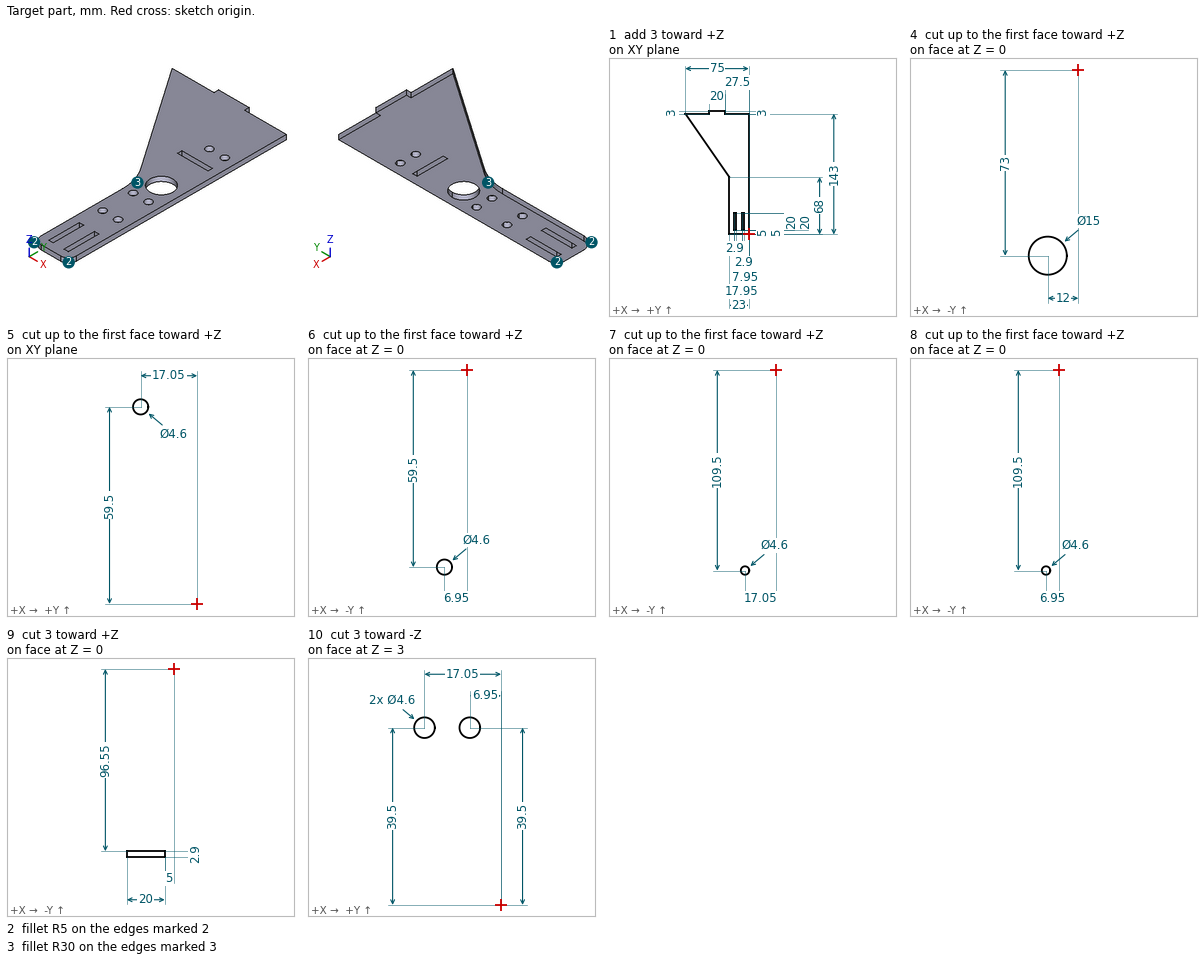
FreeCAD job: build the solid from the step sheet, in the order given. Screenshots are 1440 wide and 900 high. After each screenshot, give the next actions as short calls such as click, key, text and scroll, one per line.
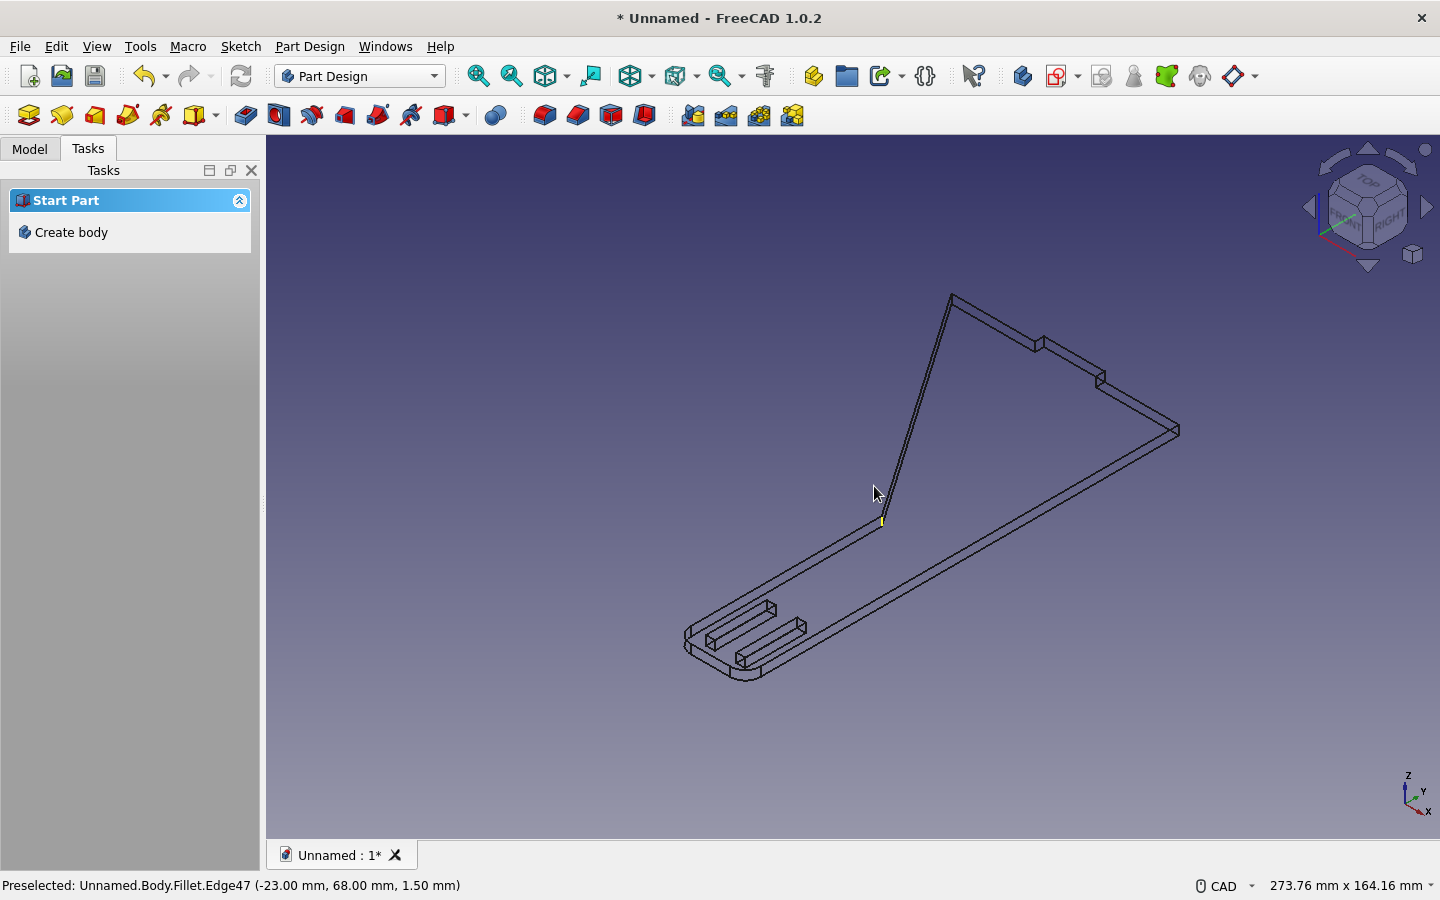
click(882, 523)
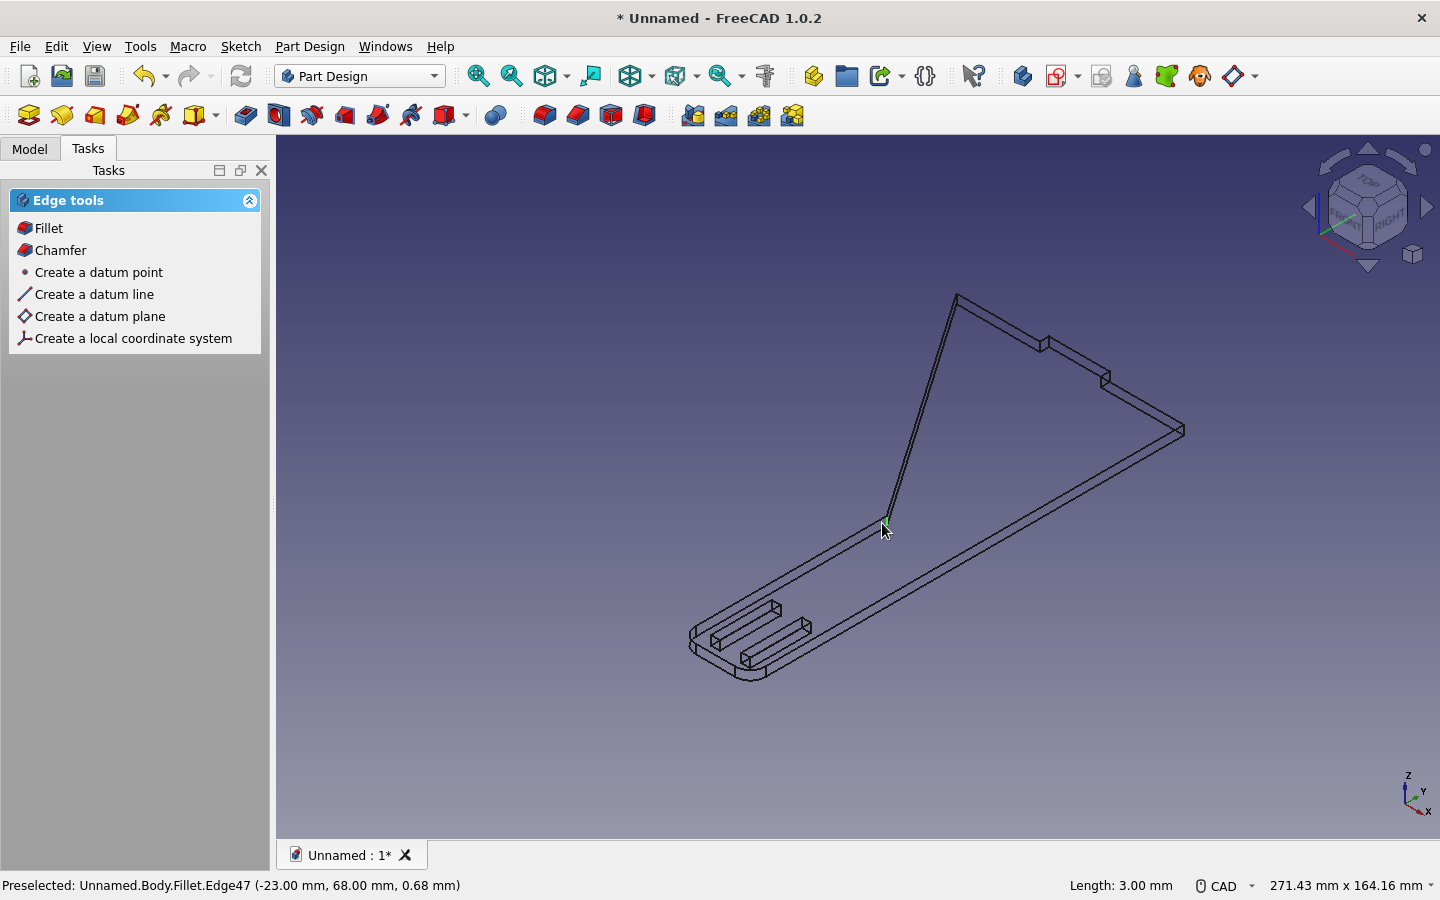
key(v)
key(1)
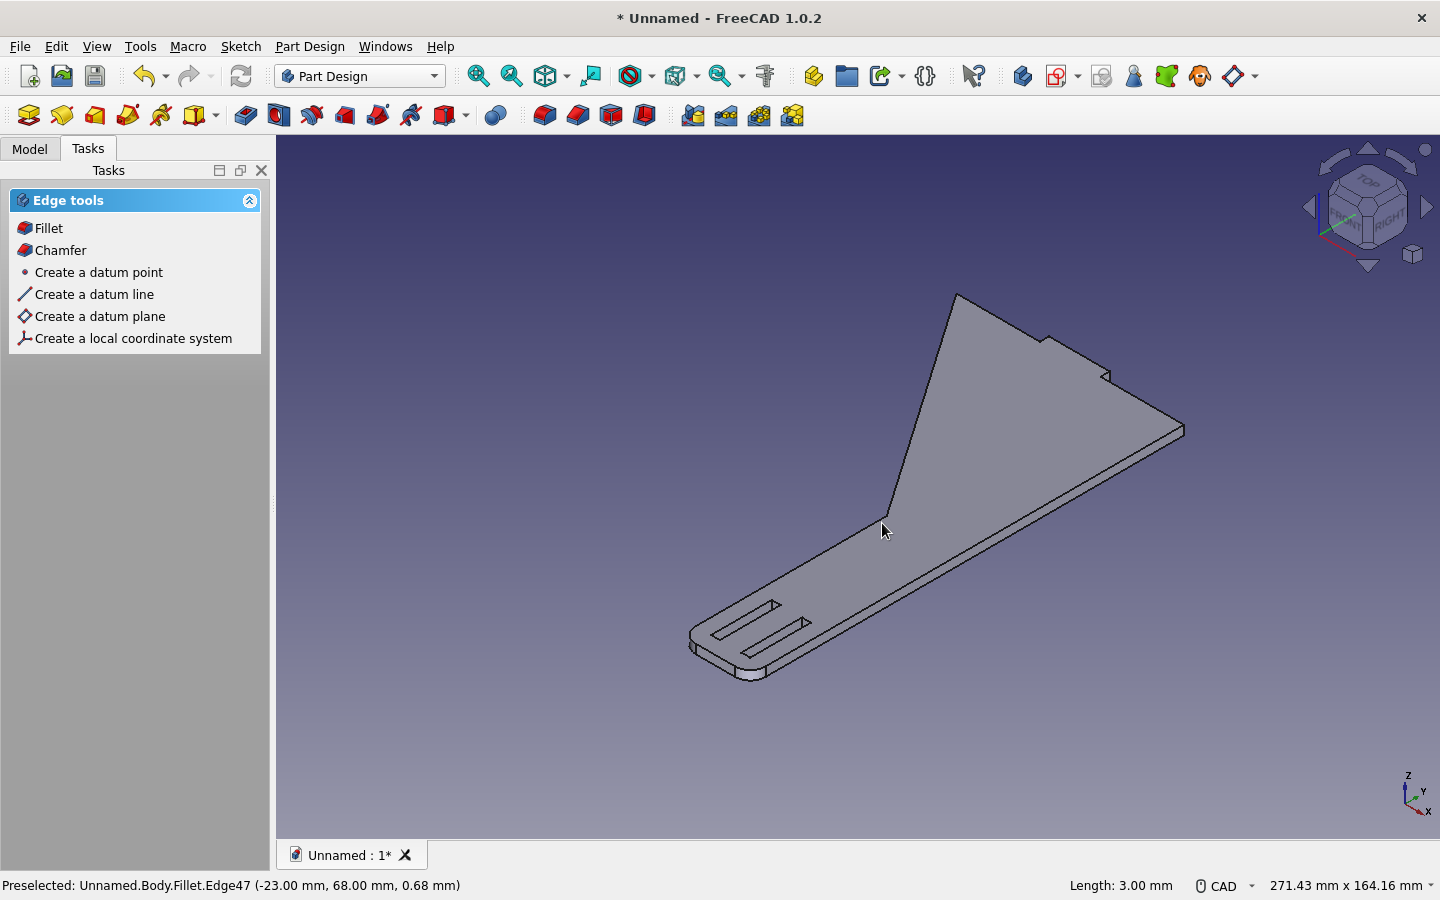
click(545, 116)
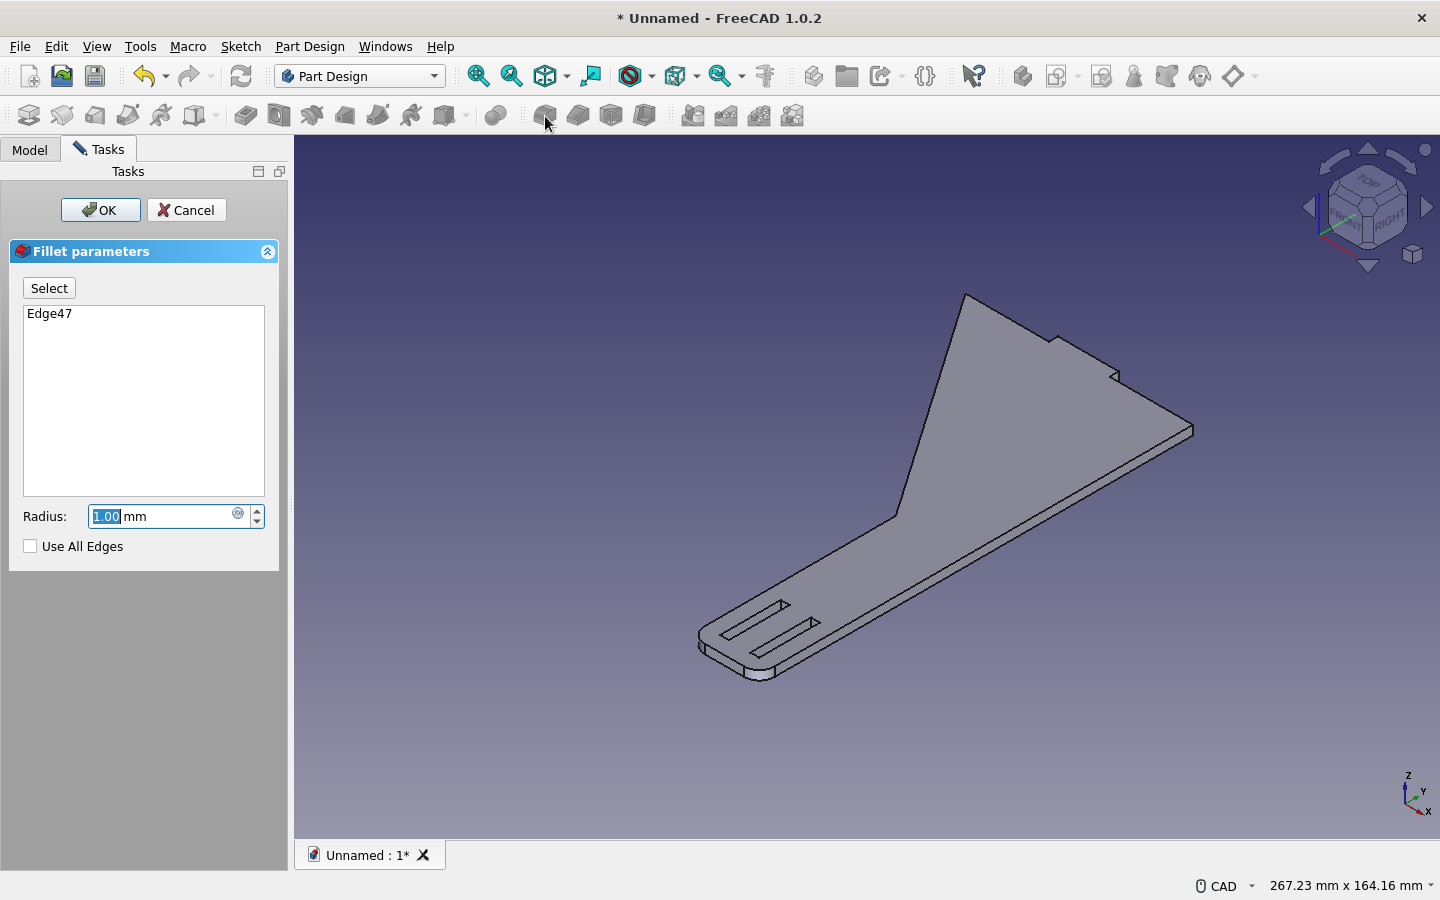
text(30)
key(Tab)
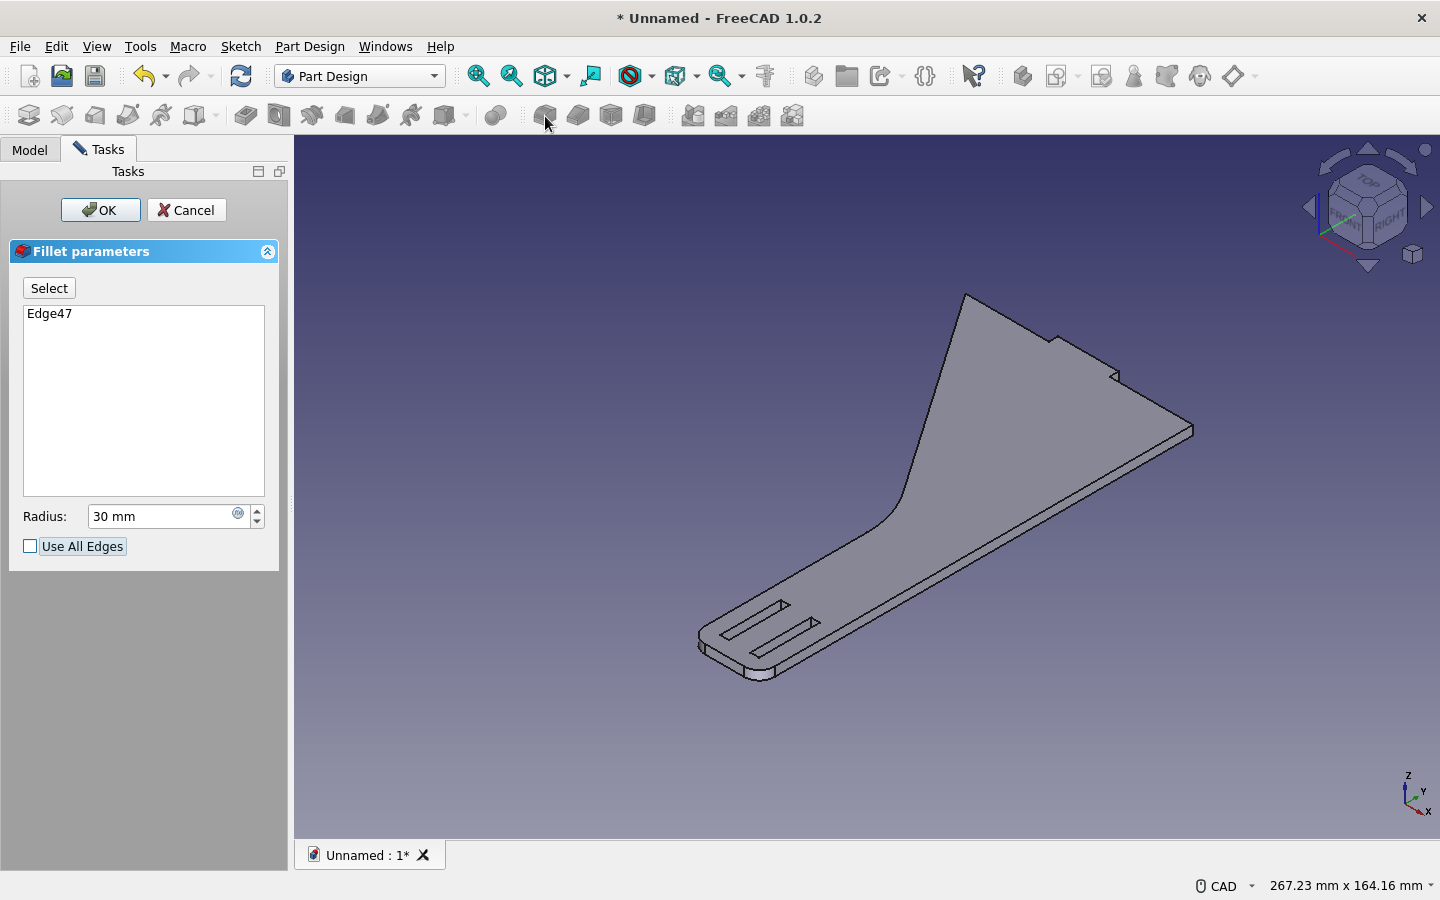
click(101, 210)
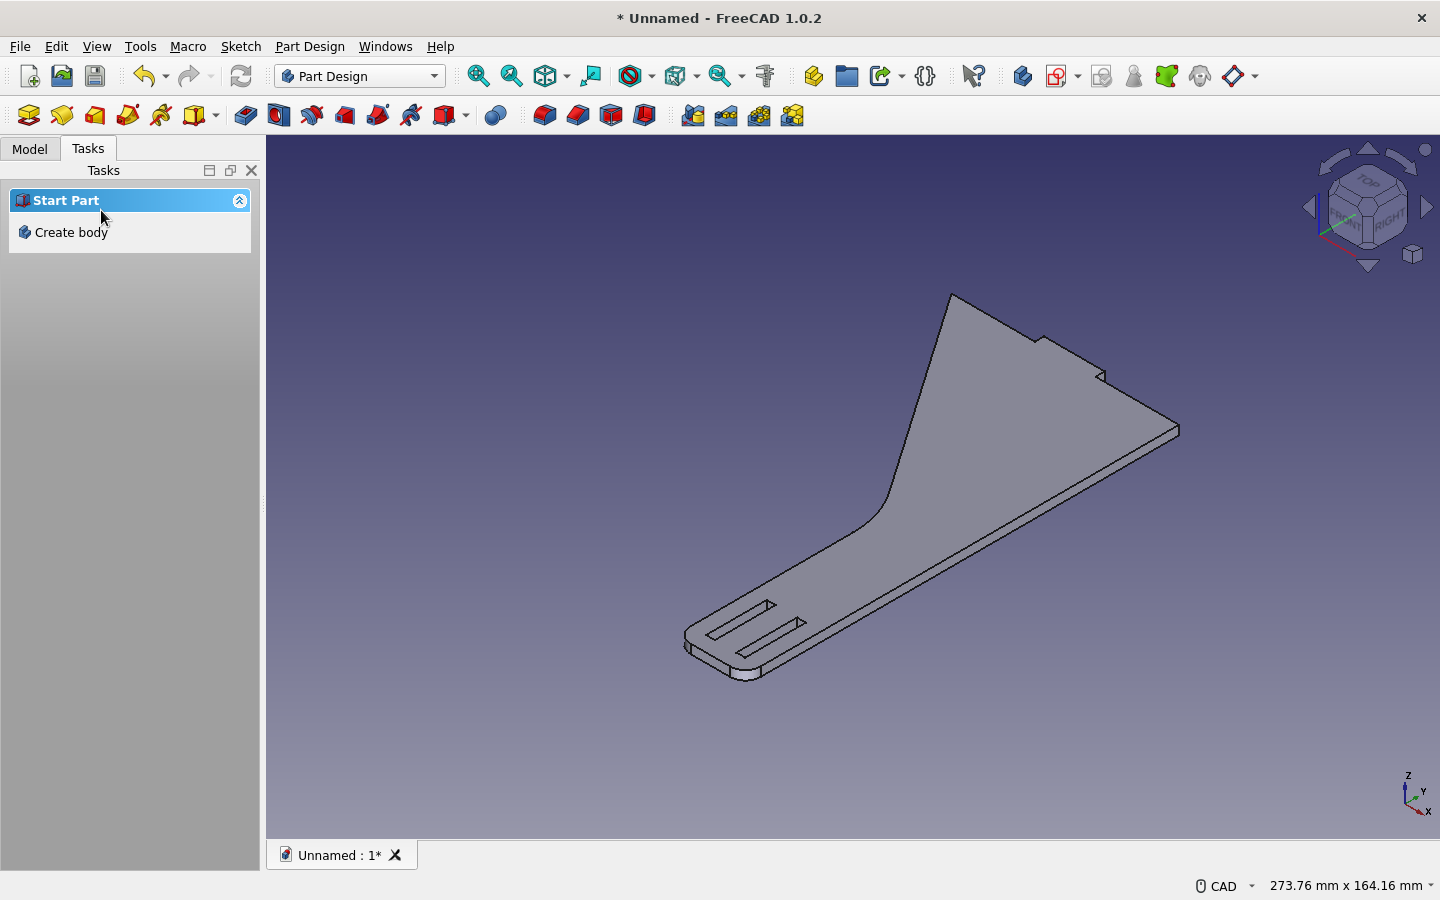
key(5)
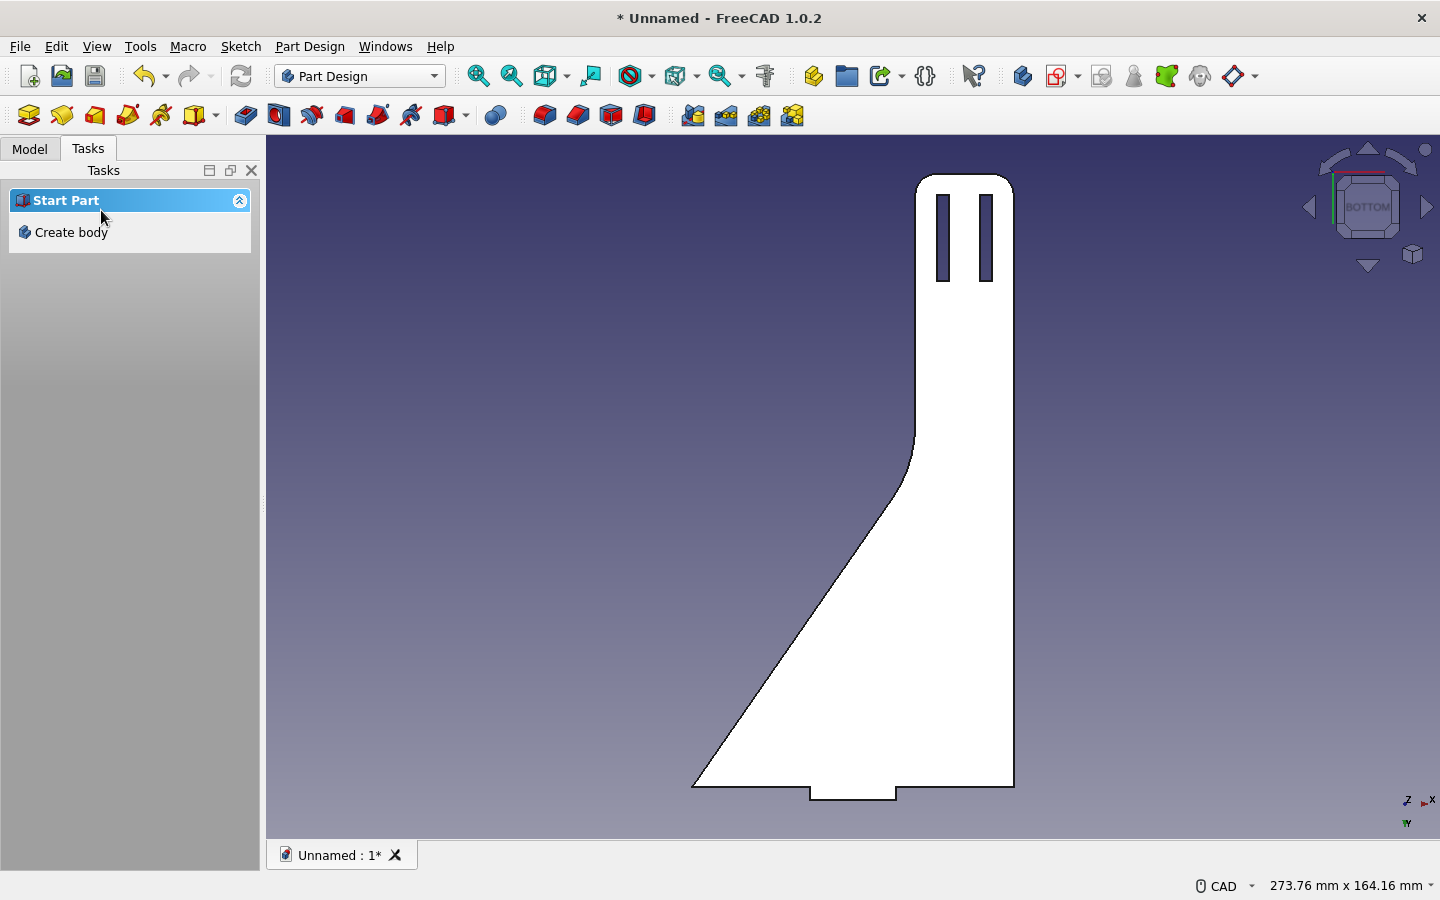
click(899, 665)